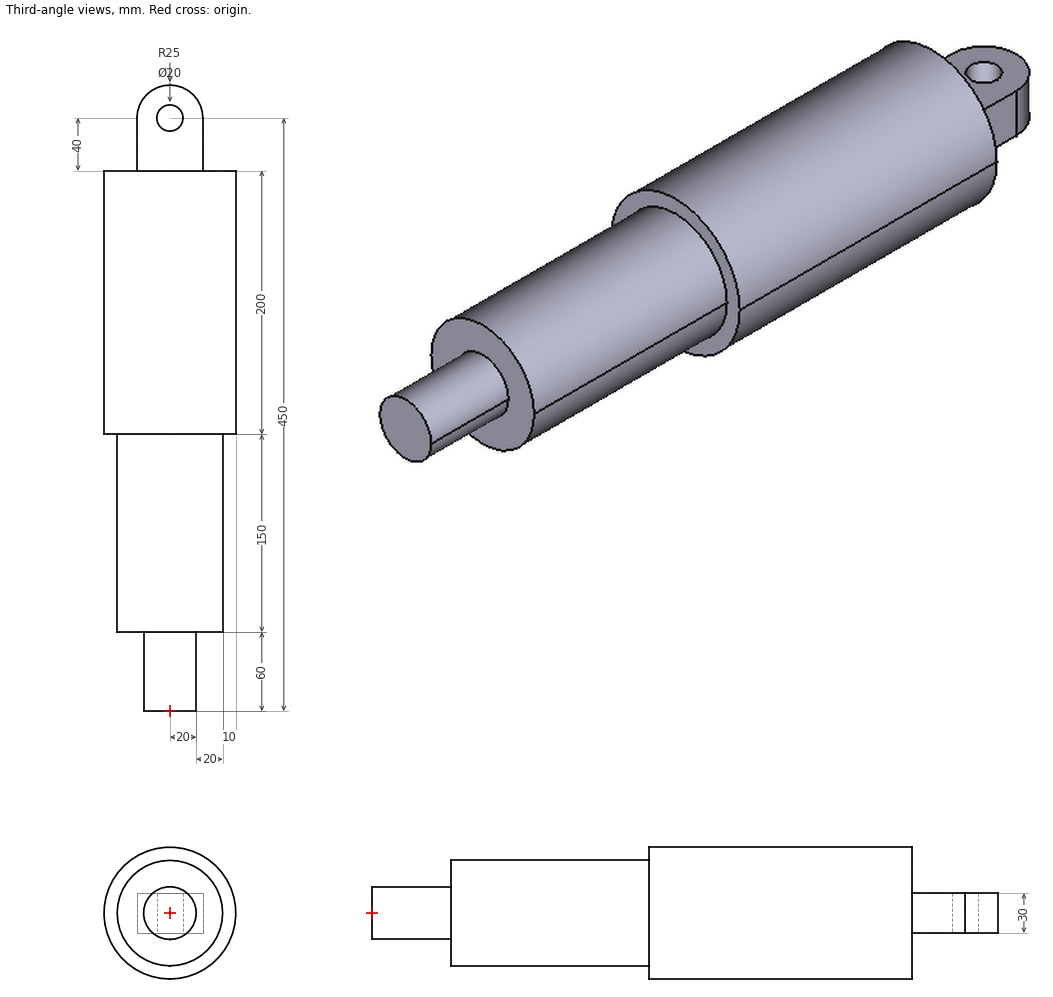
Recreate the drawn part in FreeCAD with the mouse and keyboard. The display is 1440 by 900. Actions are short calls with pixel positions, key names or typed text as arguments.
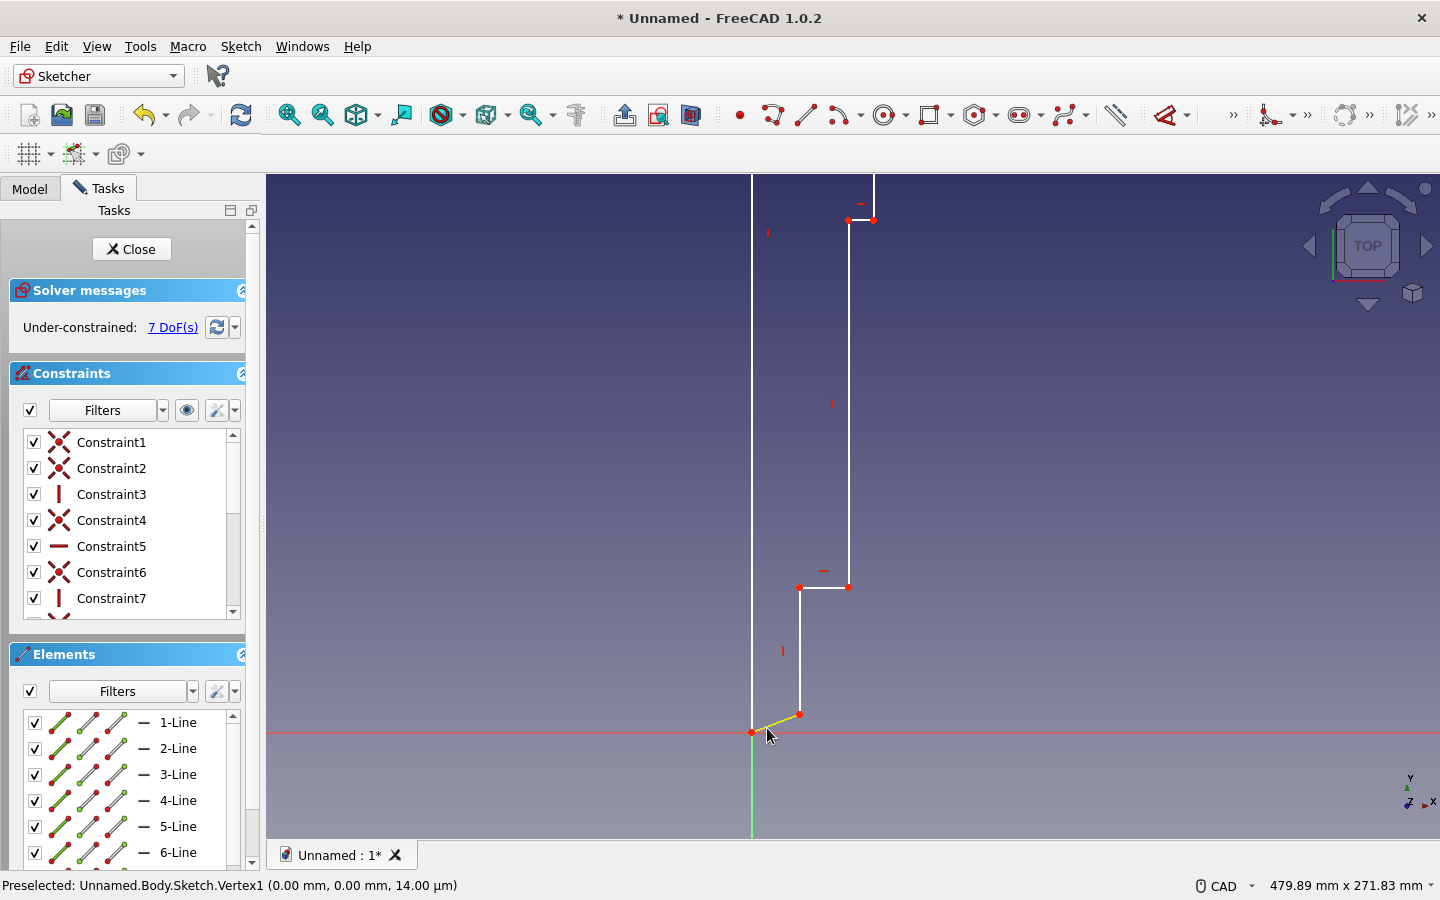
click(766, 727)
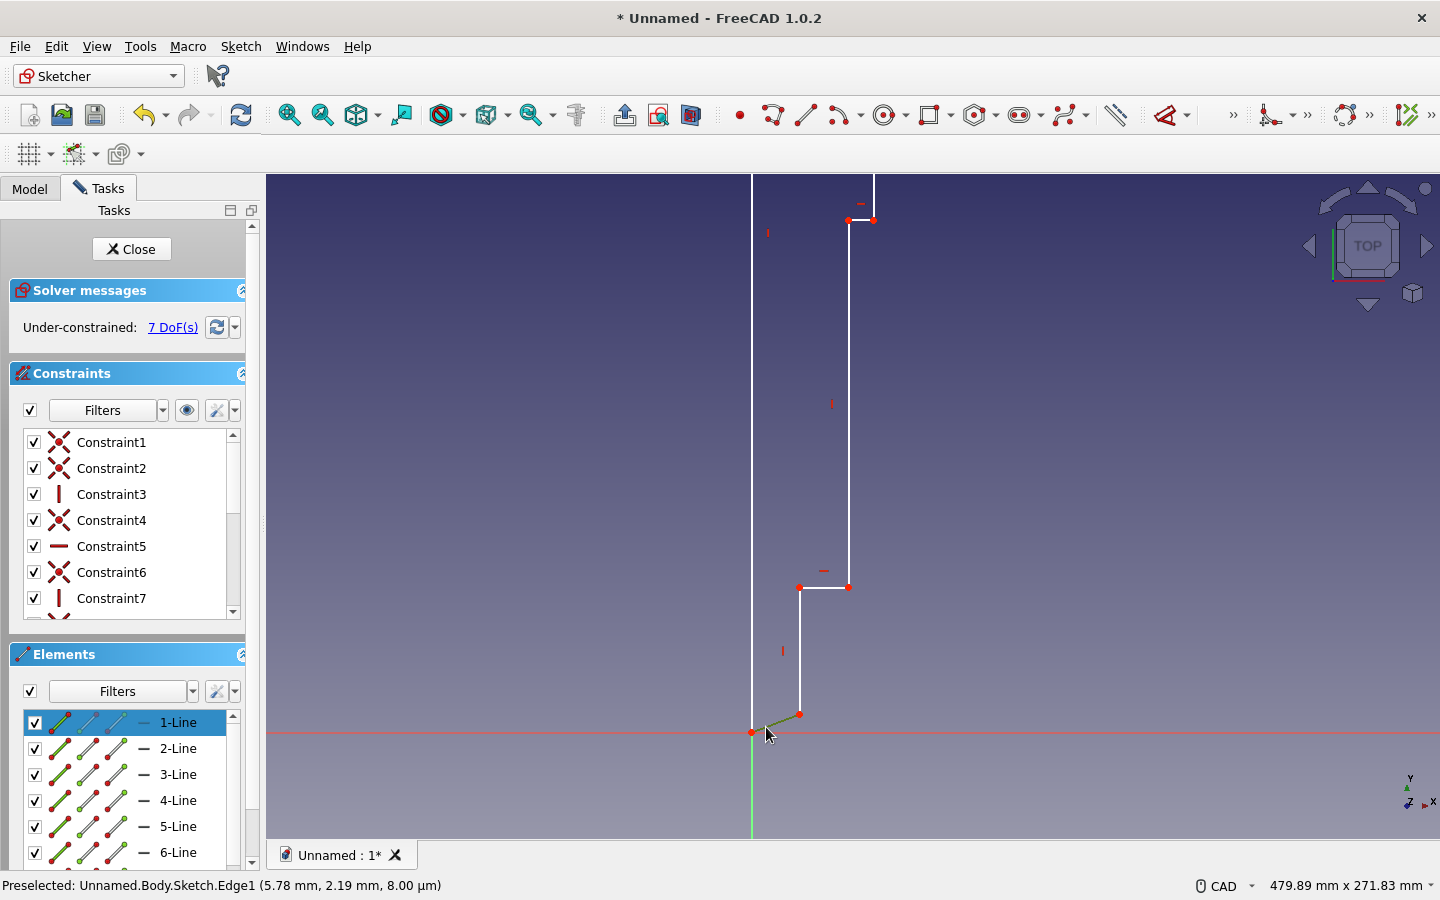
key(h)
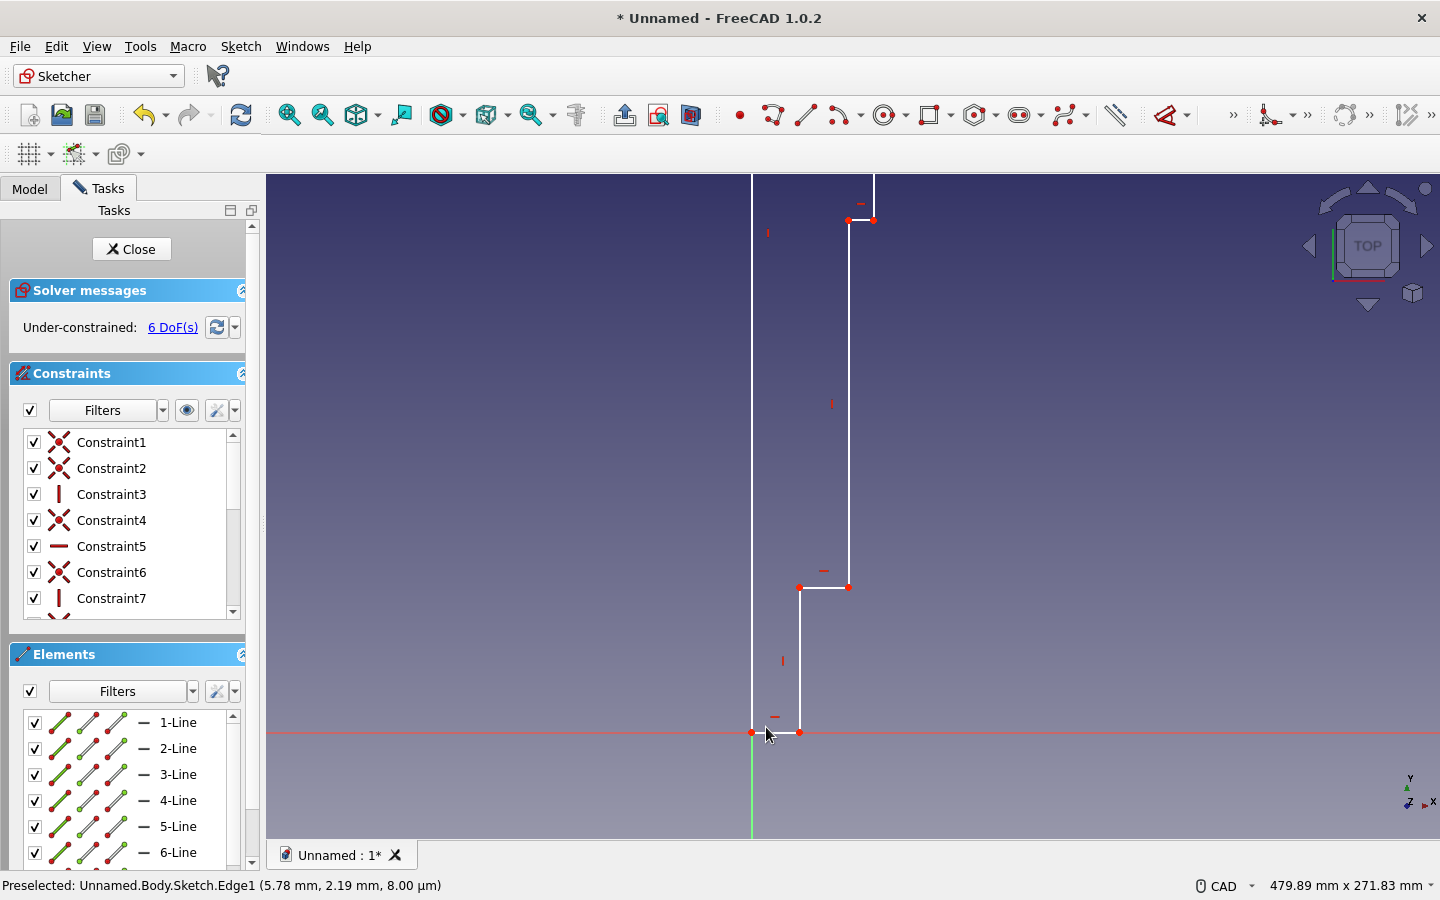
click(1164, 116)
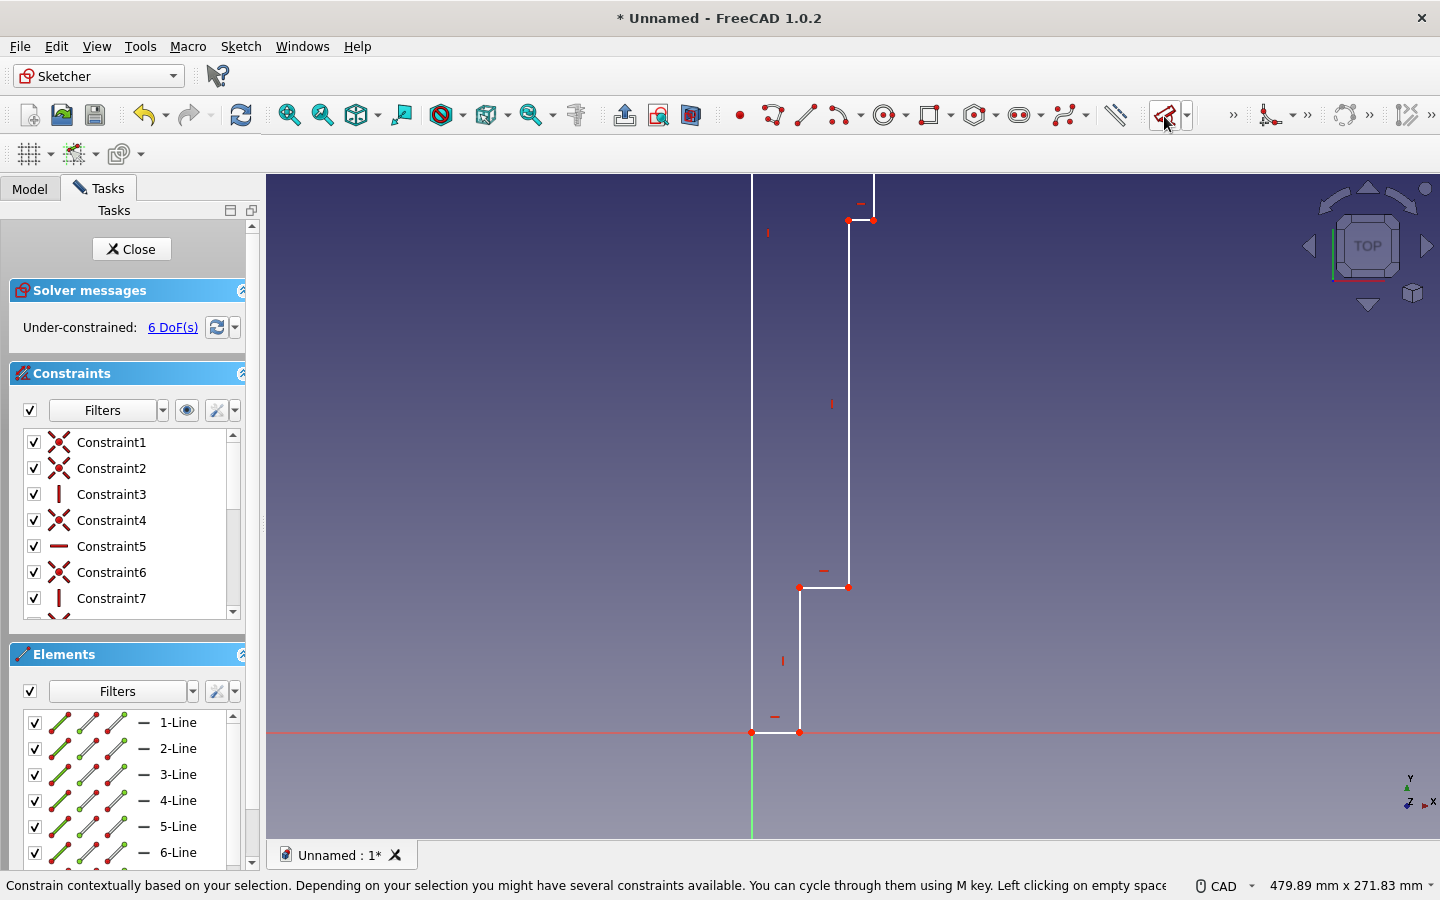
click(766, 733)
click(776, 767)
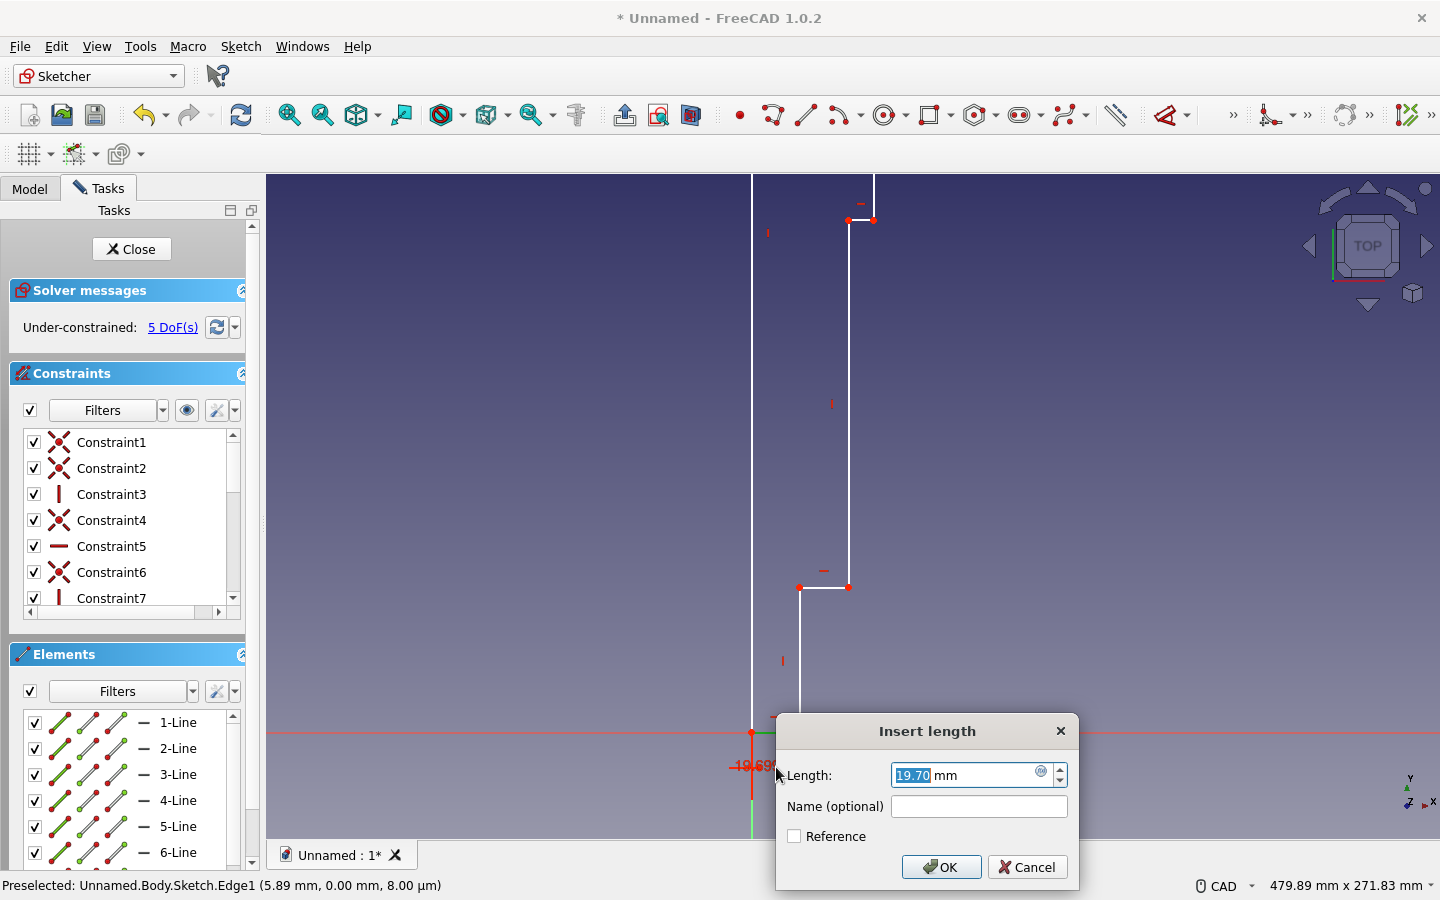
text(20)
key(Return)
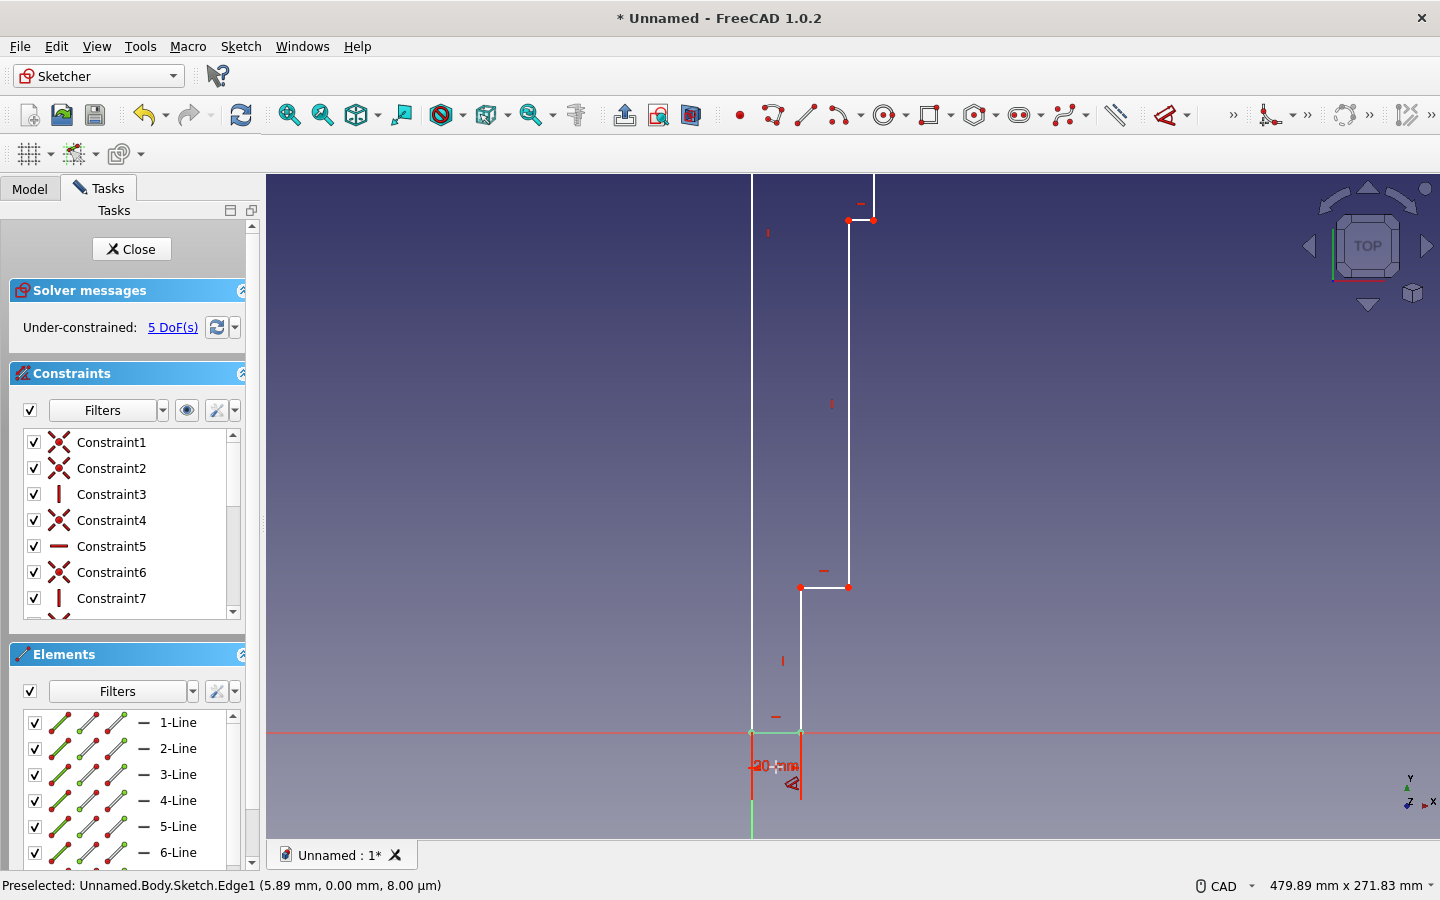
click(801, 689)
click(767, 660)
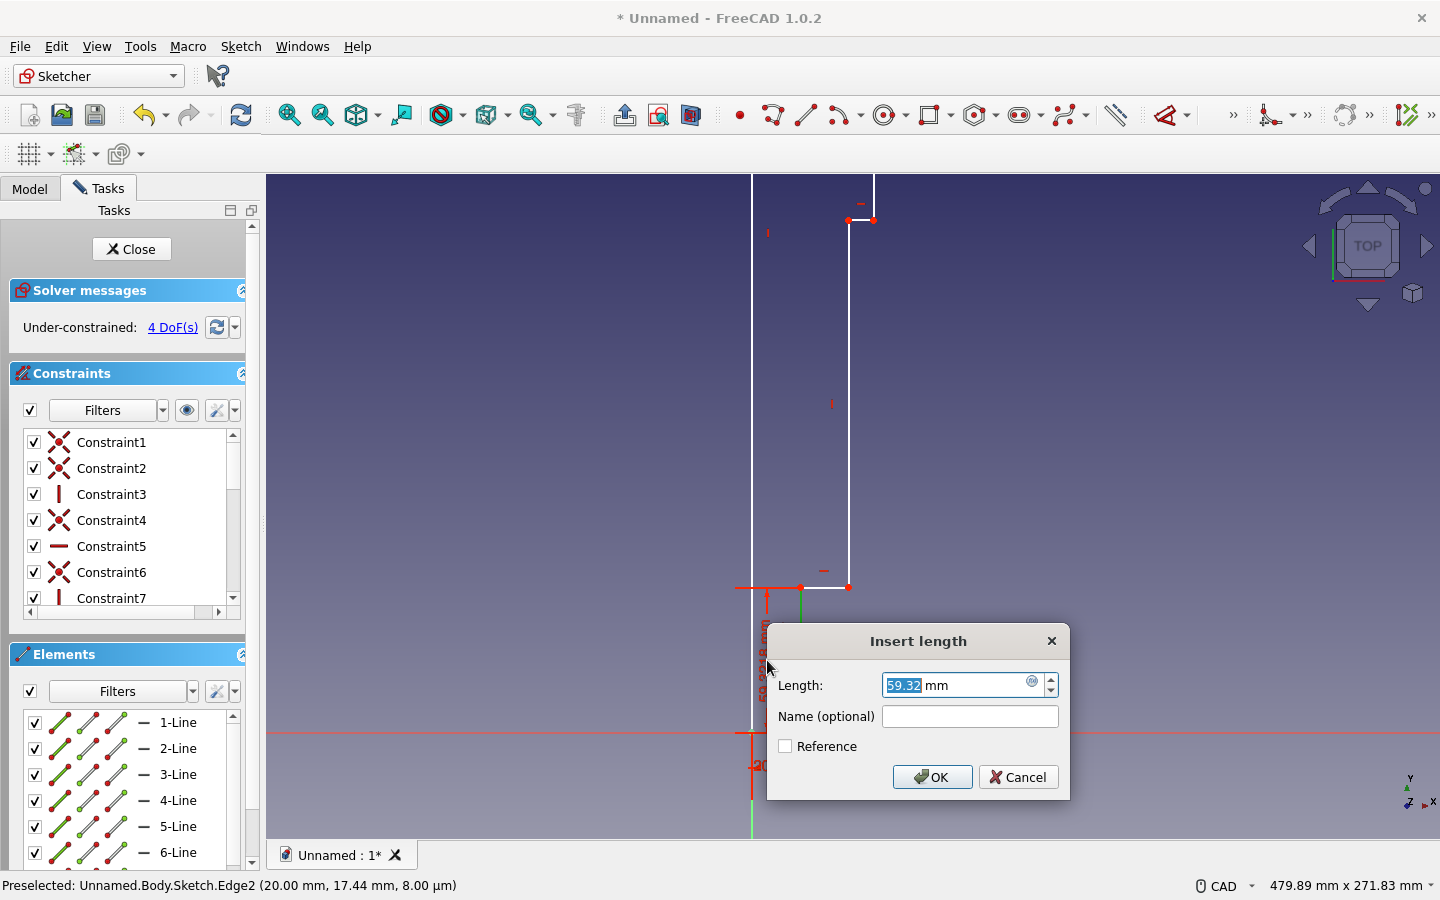
text(60)
key(Return)